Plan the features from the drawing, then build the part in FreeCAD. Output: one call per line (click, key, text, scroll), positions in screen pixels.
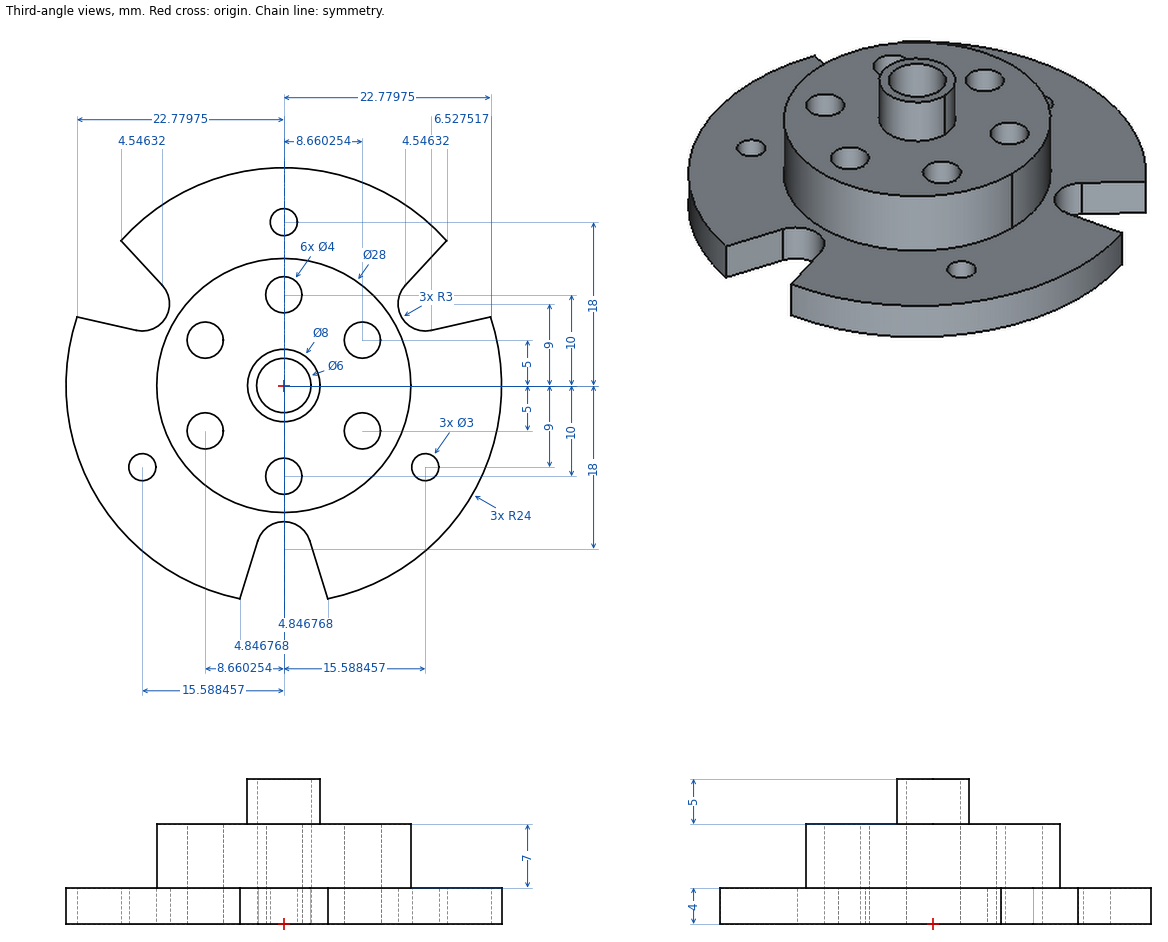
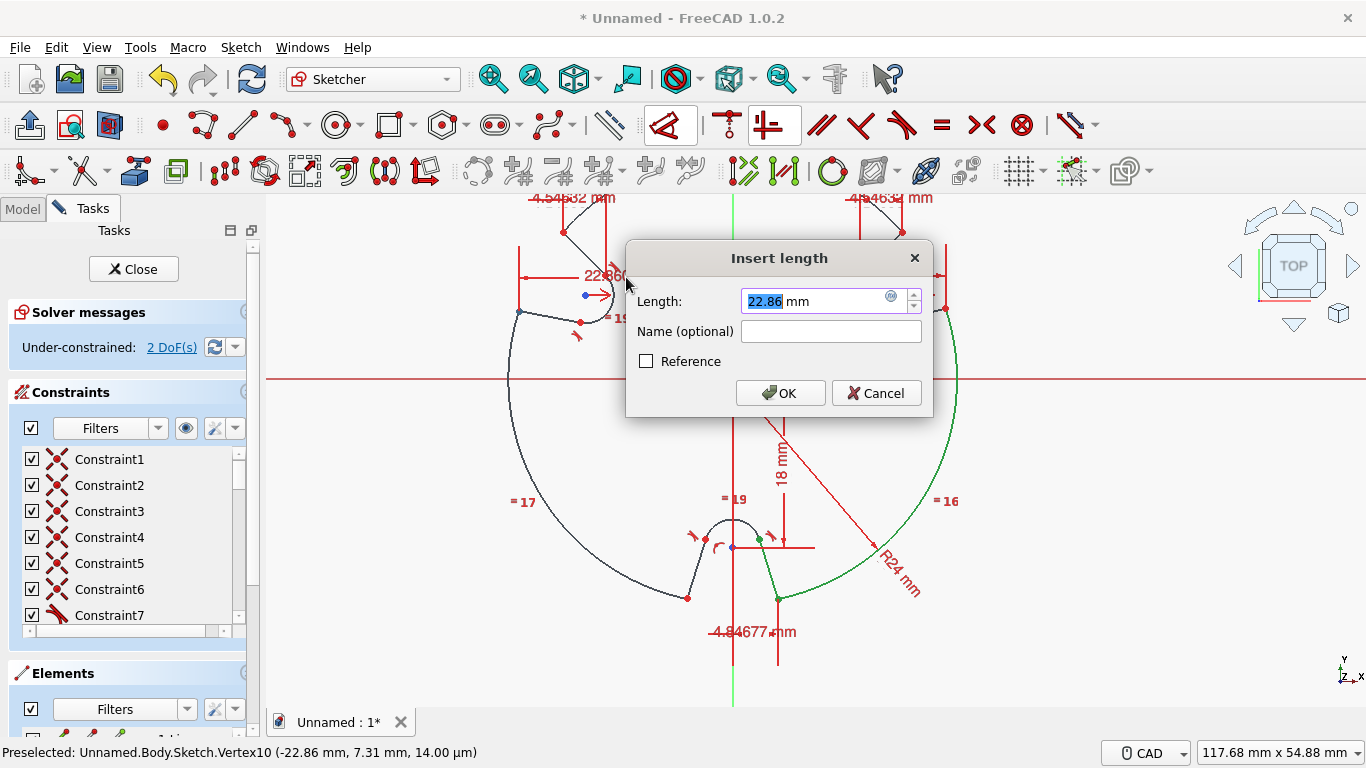
text(22.77975)
key(Return)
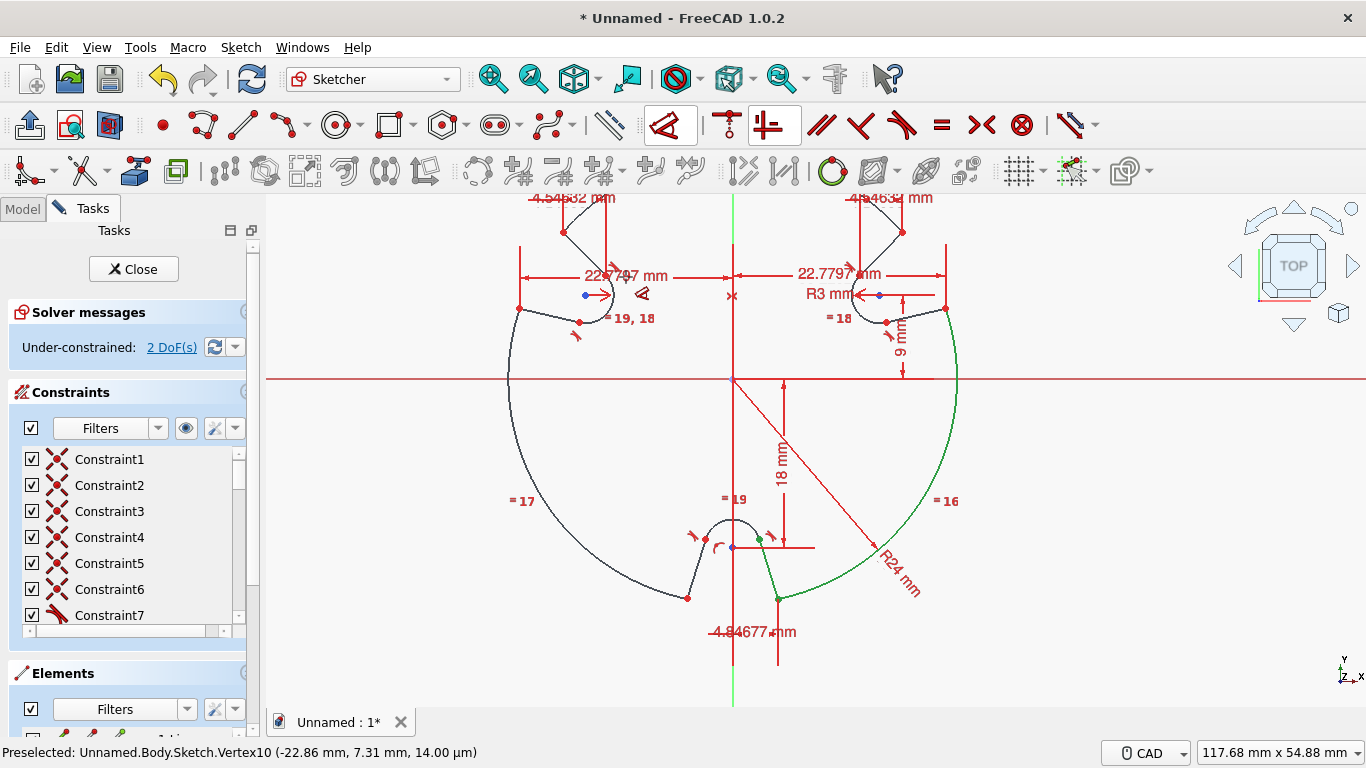
click(687, 599)
click(710, 345)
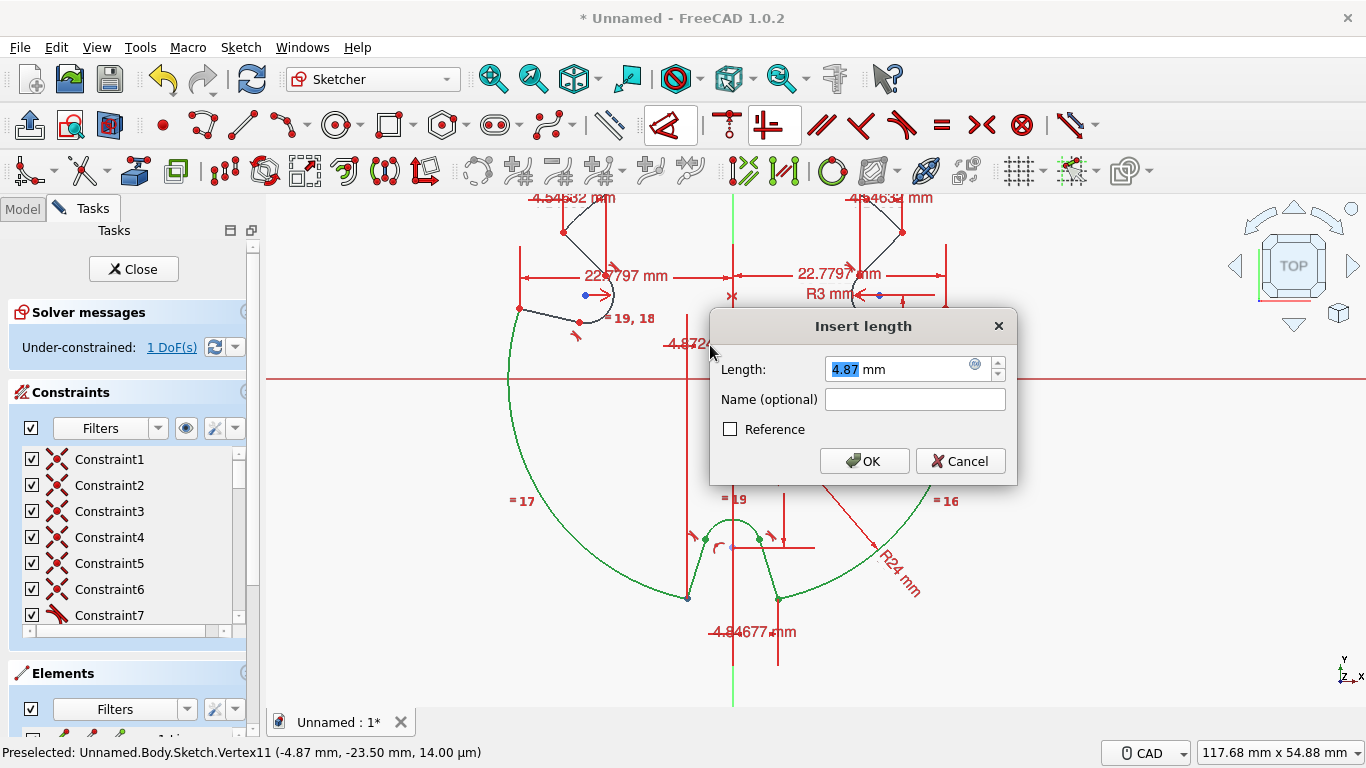
text(4.846768)
key(Return)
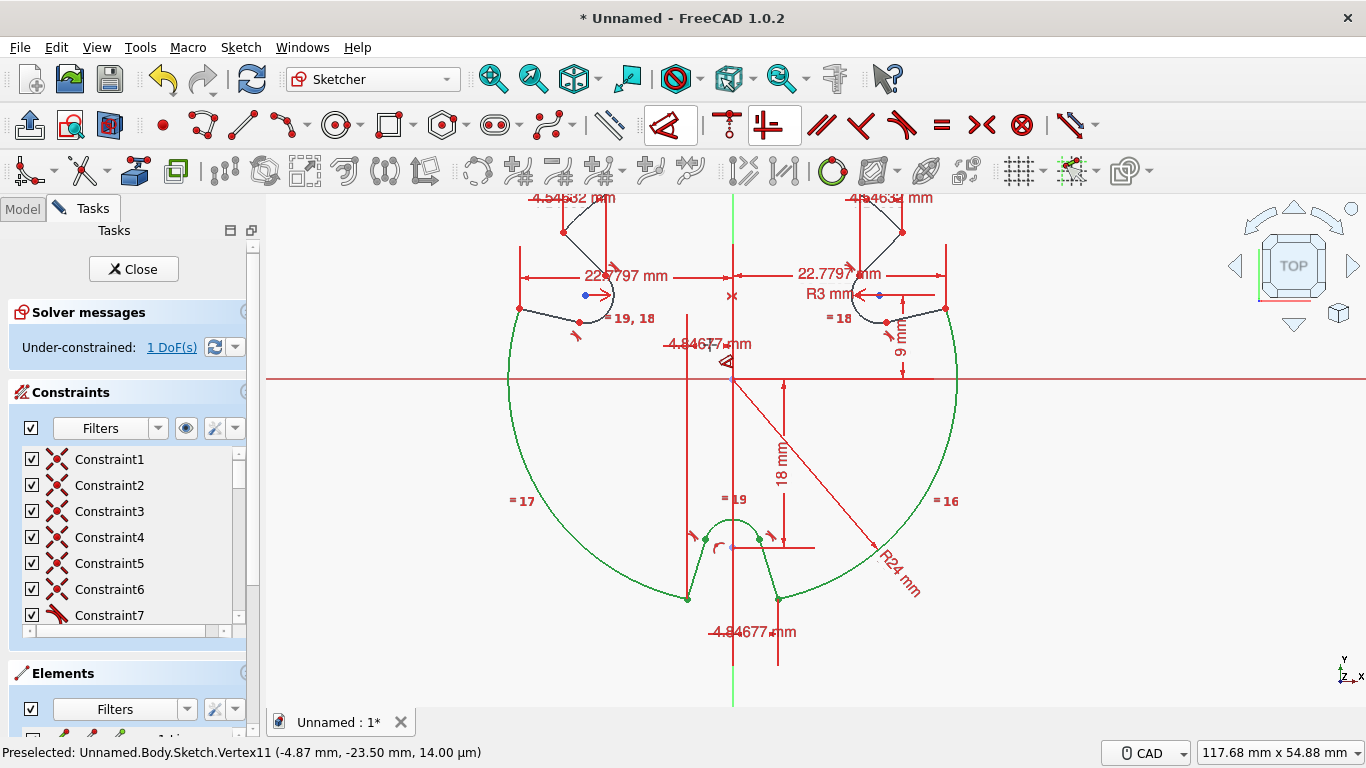
click(928, 313)
click(916, 275)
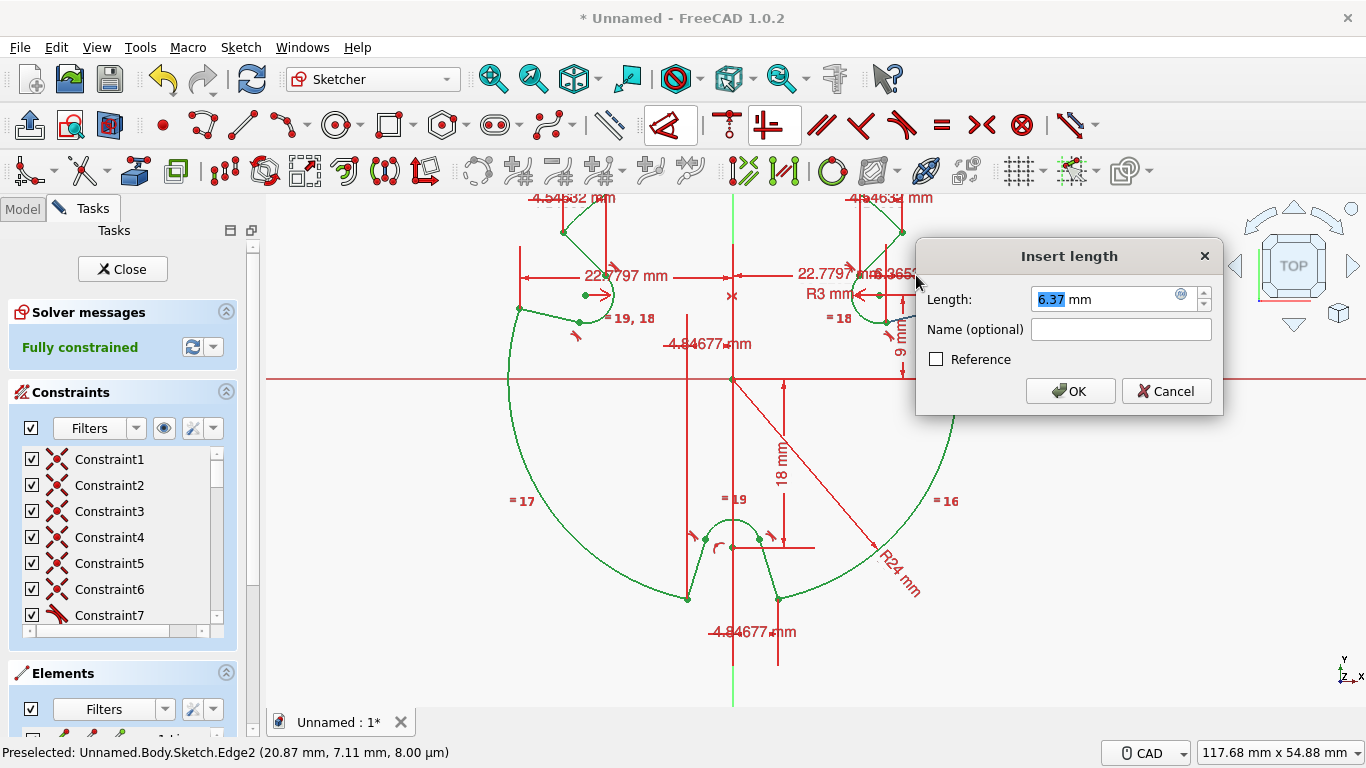
text(6.527517)
key(Return)
key(Escape)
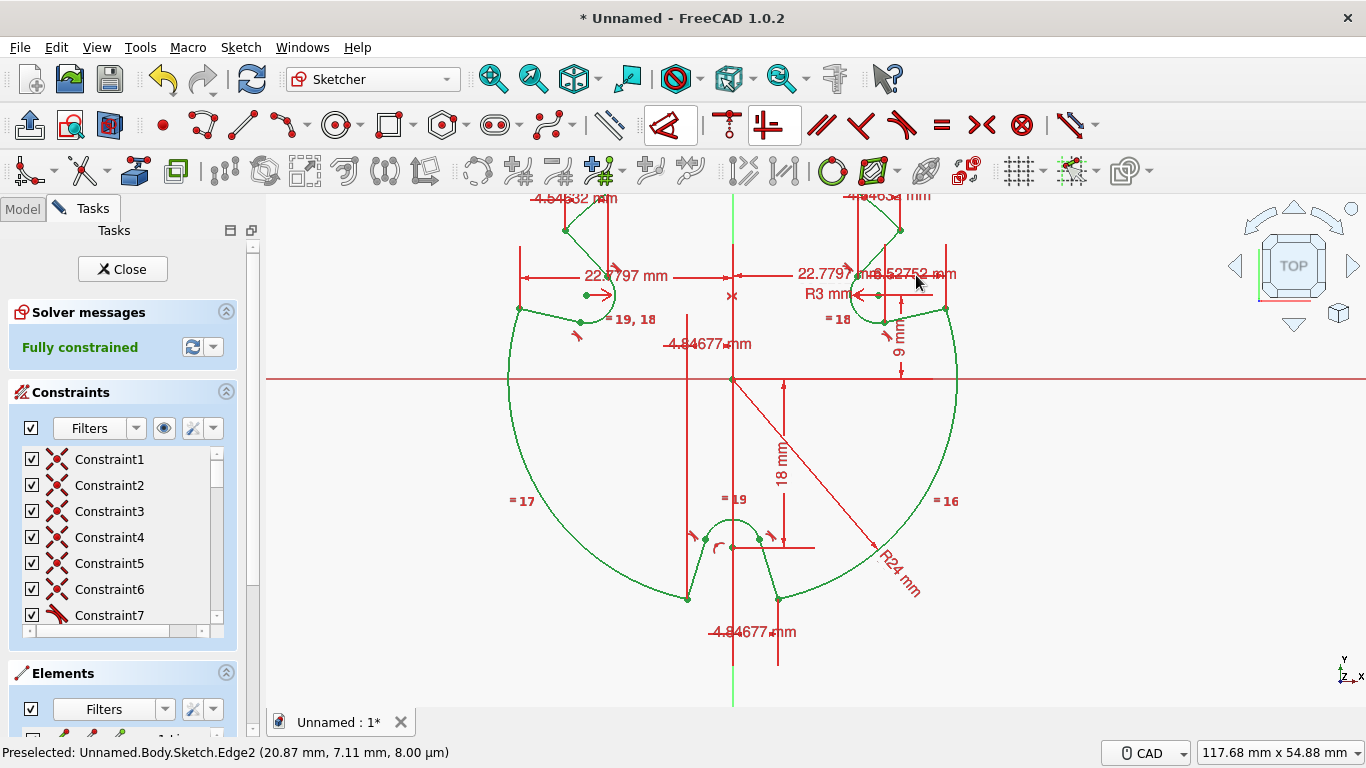
click(123, 269)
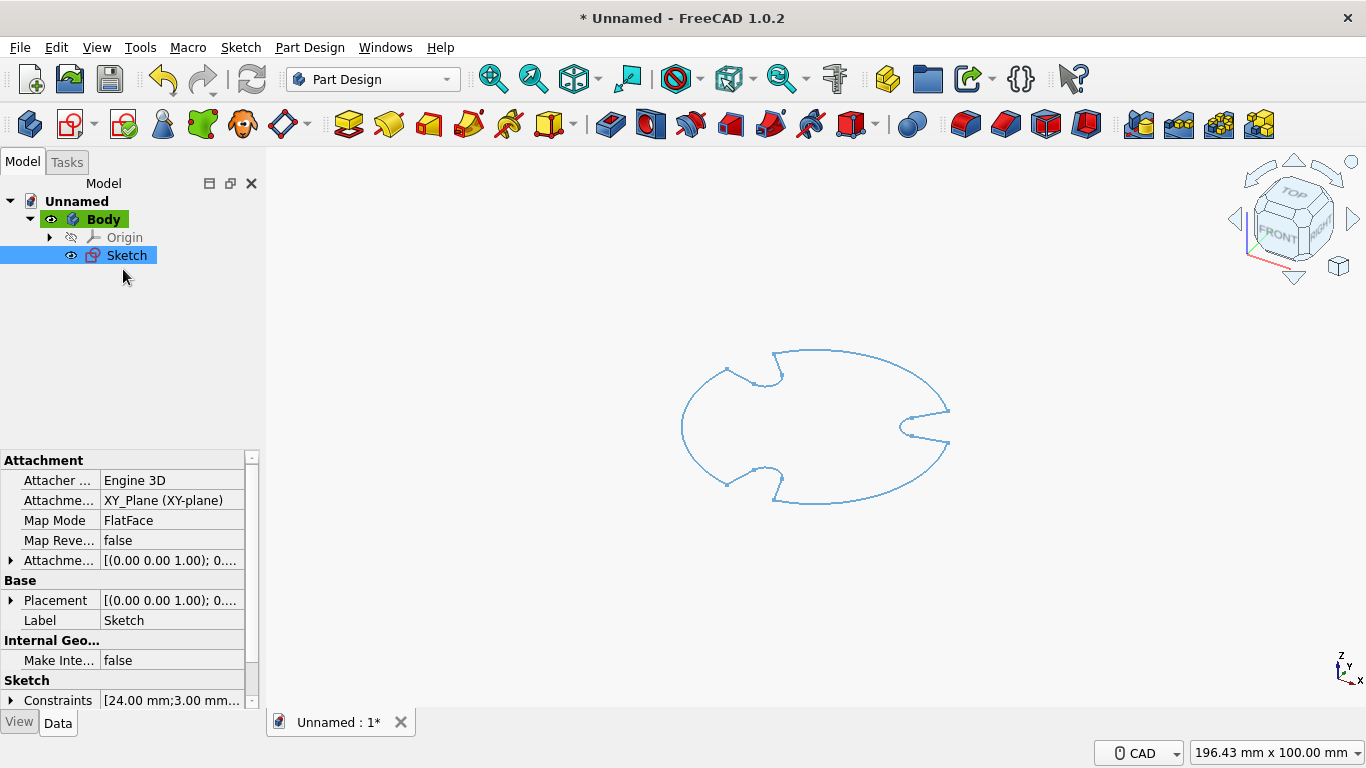
click(350, 124)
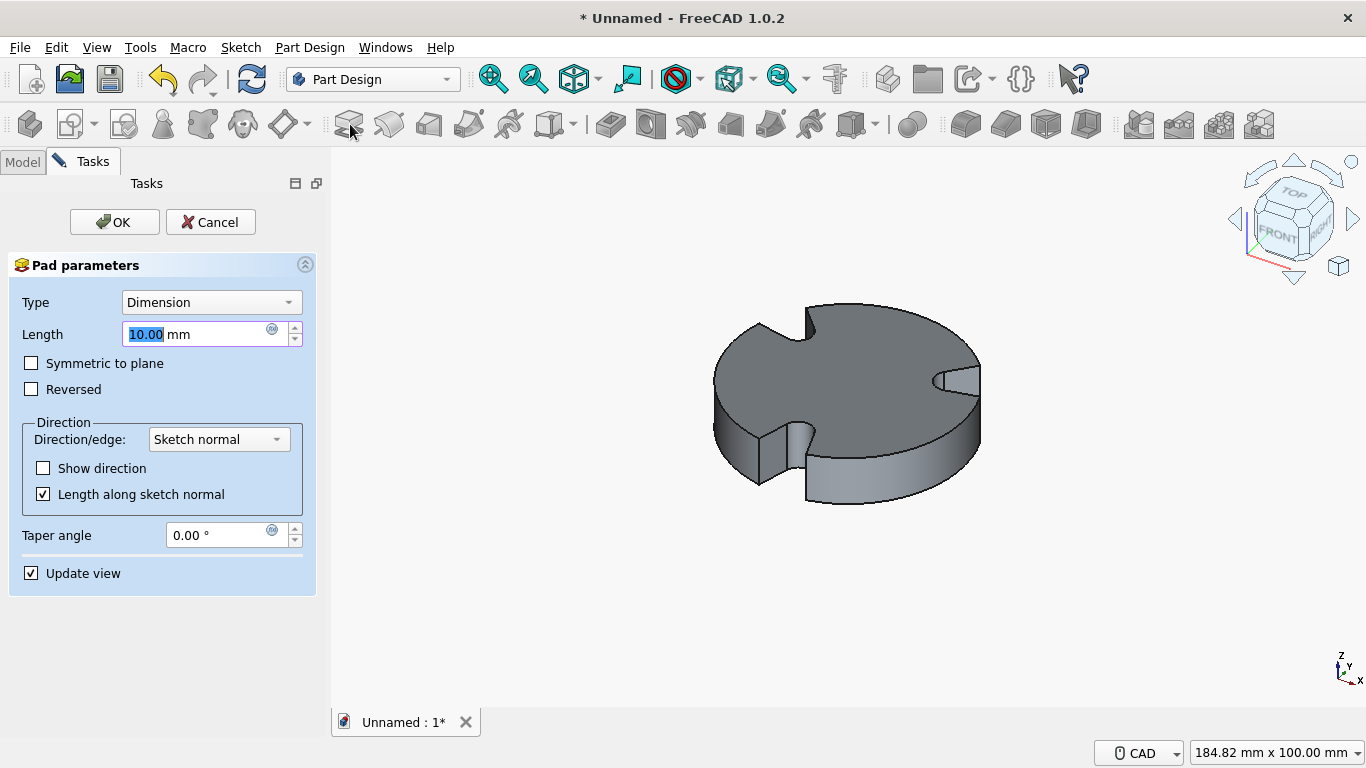
text(4)
key(Tab)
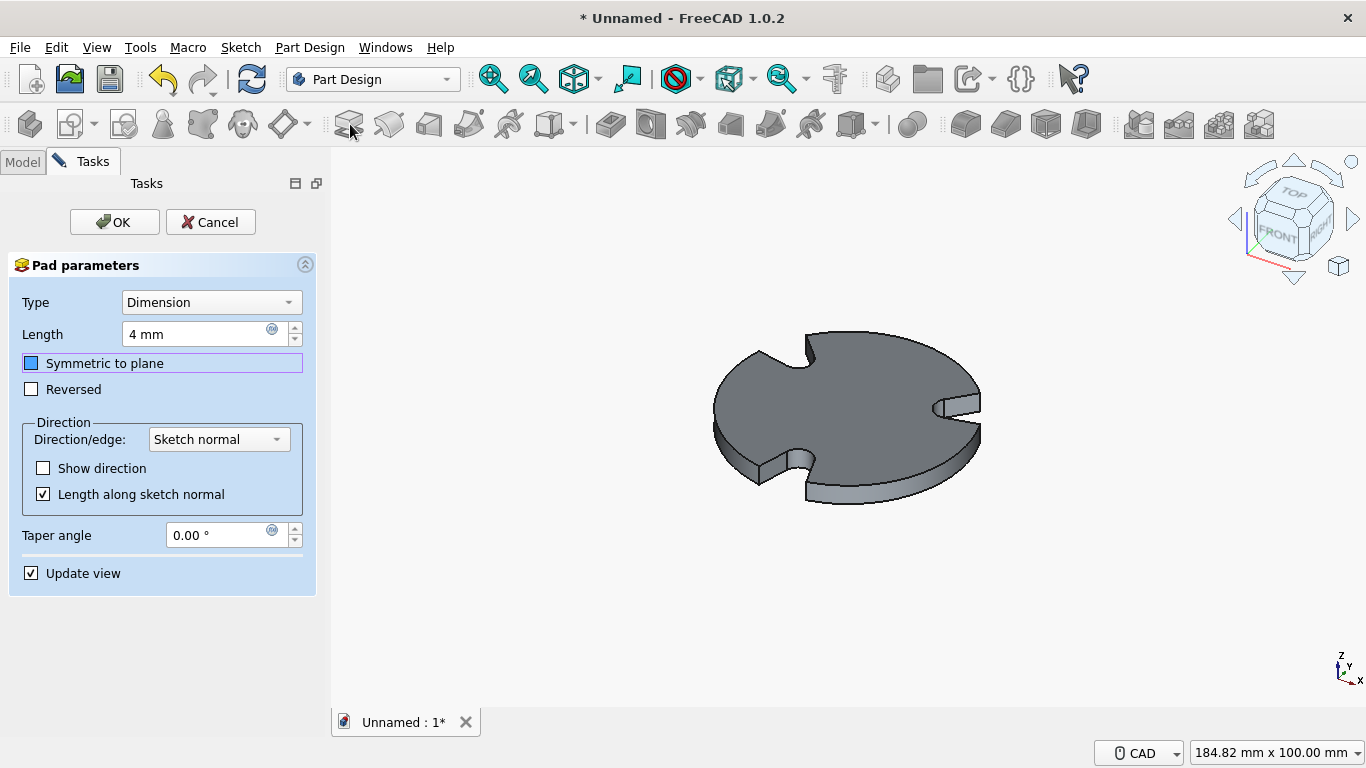
click(115, 222)